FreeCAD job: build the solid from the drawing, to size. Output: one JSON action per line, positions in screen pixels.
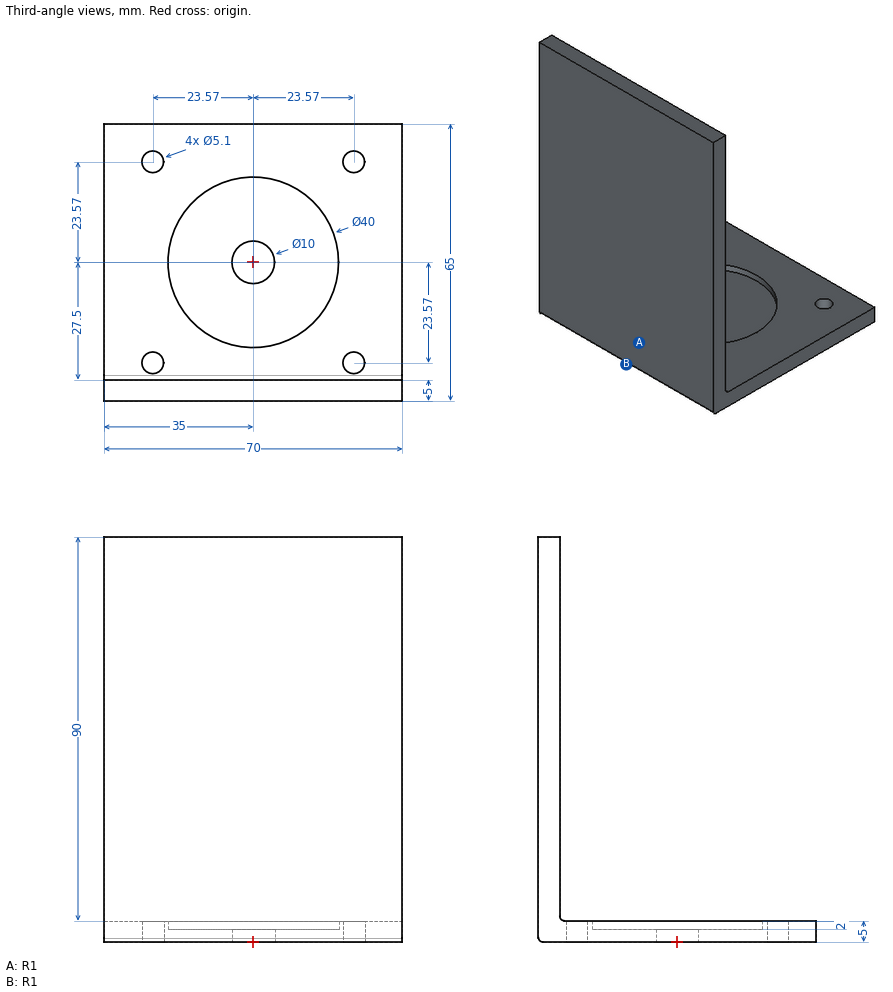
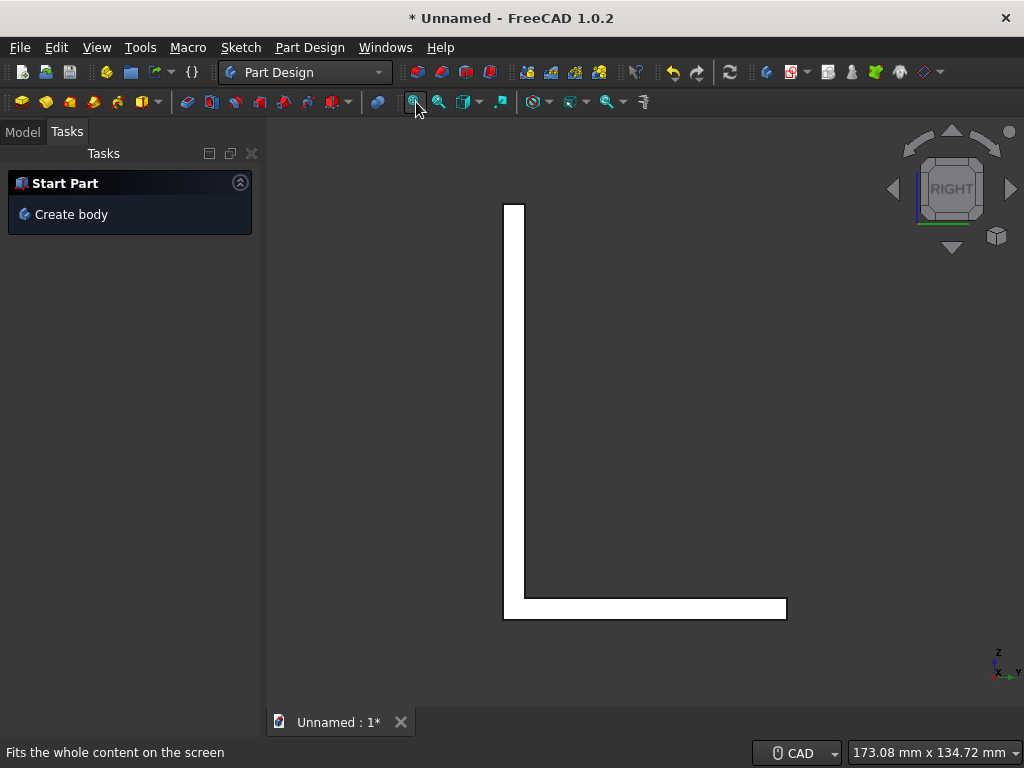
{"action": "key", "text": "5"}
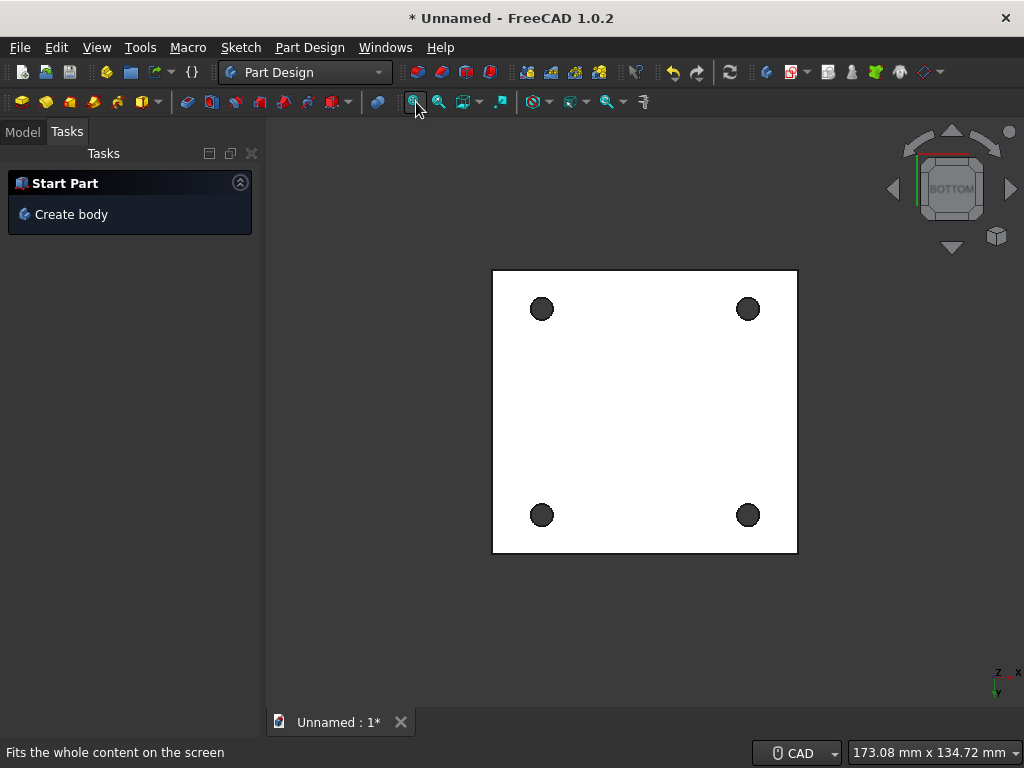
{"action": "key", "text": "4"}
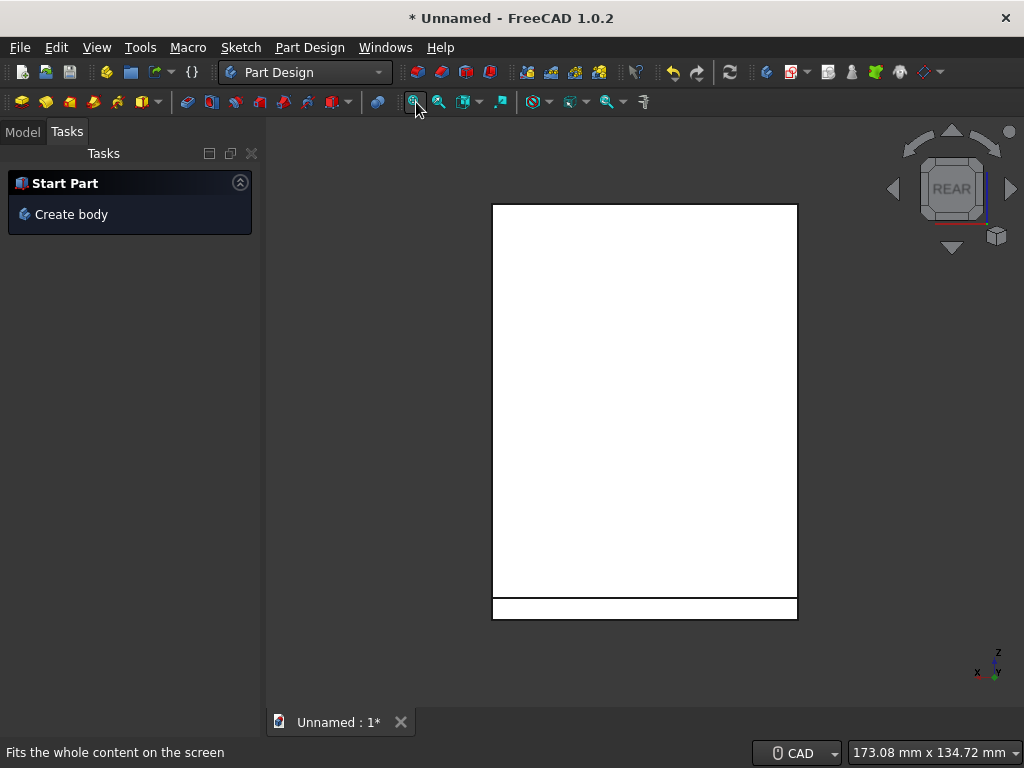
{"action": "key", "text": "6"}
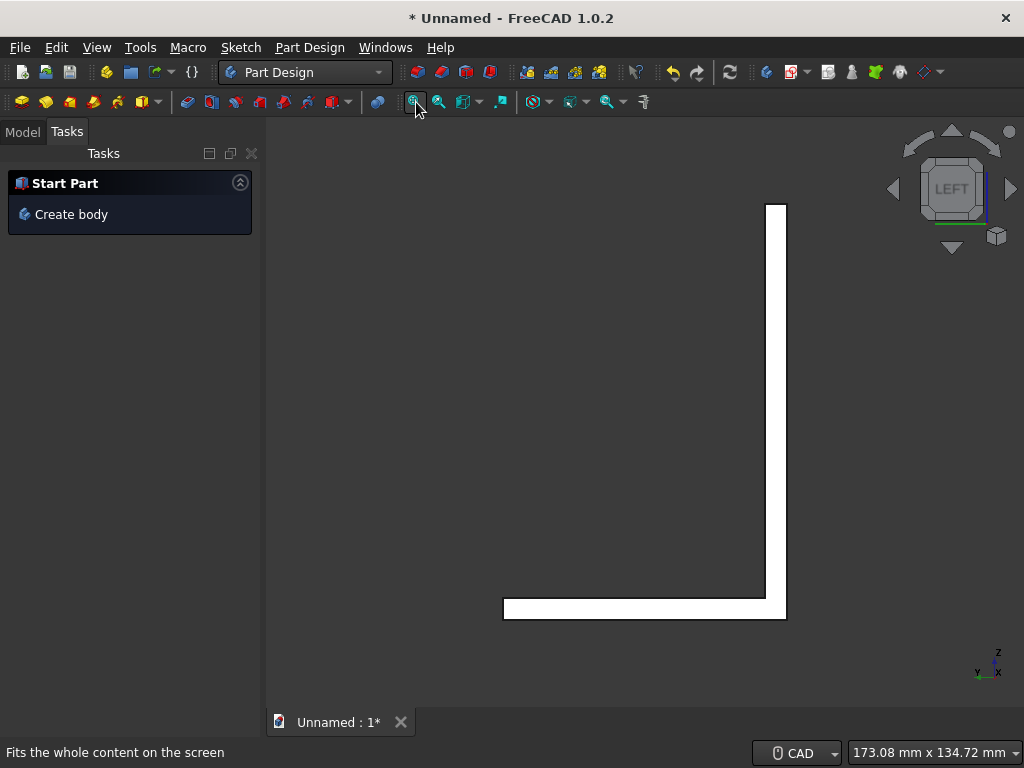
{"action": "key", "text": "v 3"}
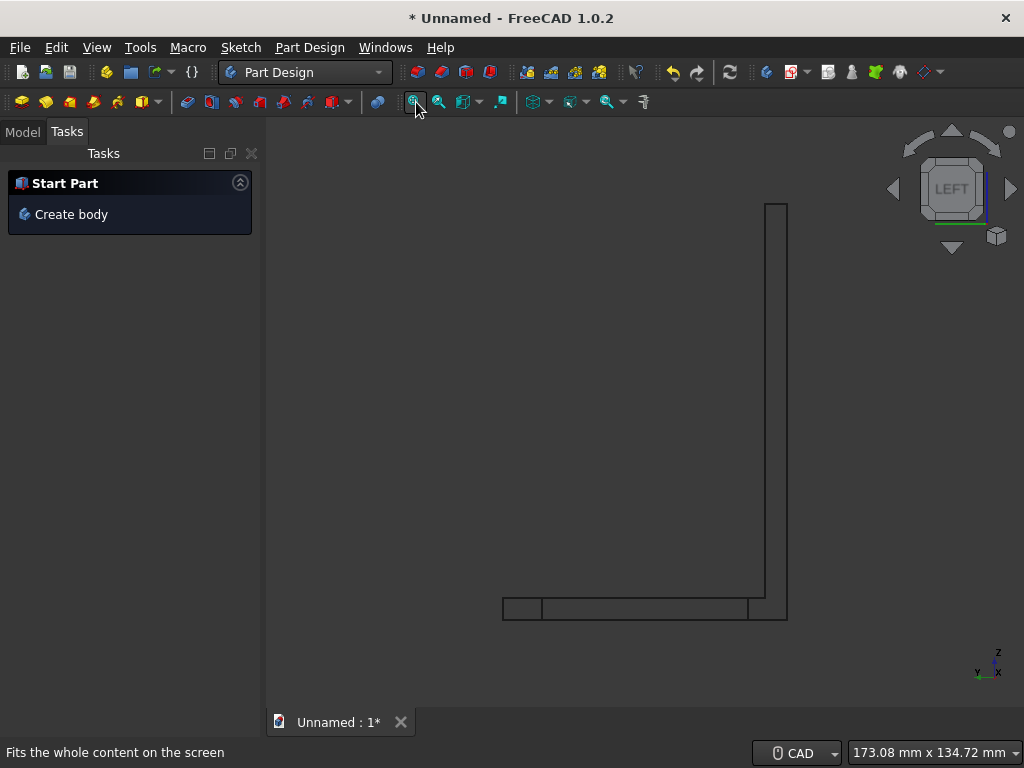
{"action": "key", "text": "0"}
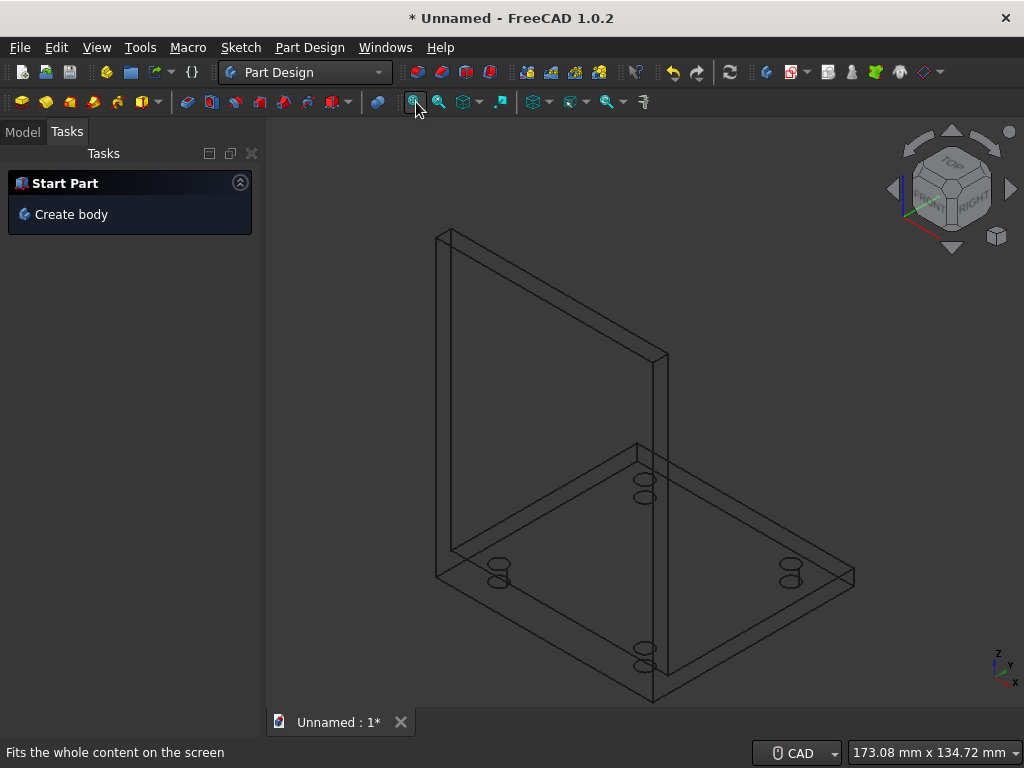
{"action": "left_click", "coordinate": [560, 612]}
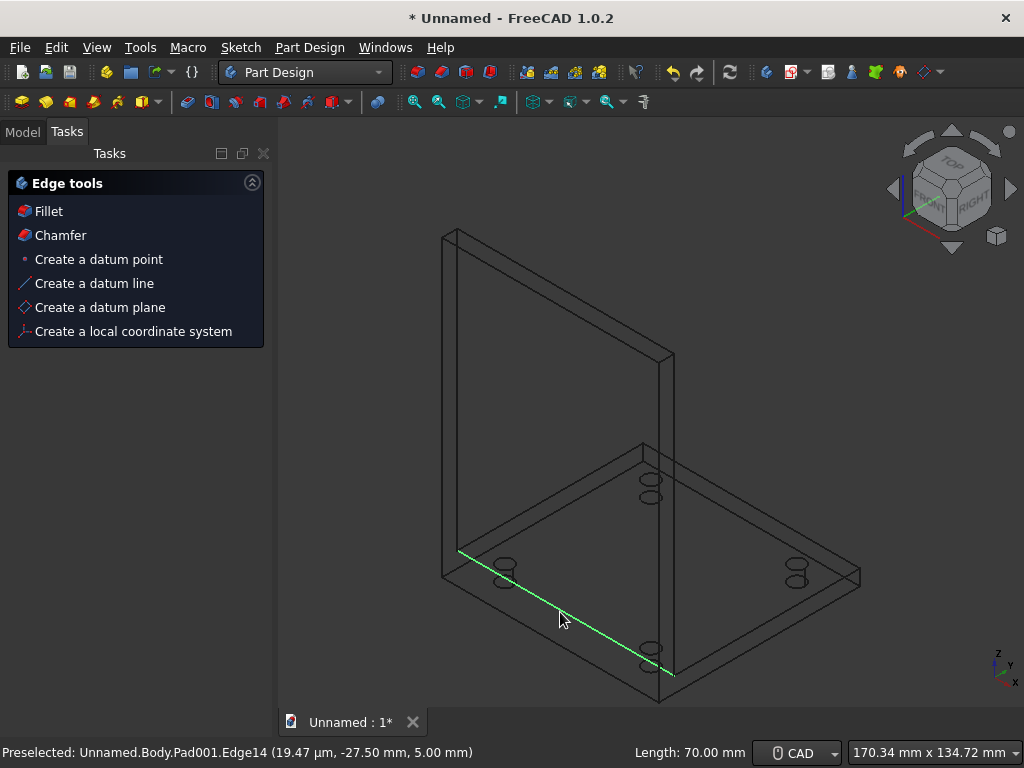
{"action": "key", "text": "v 1"}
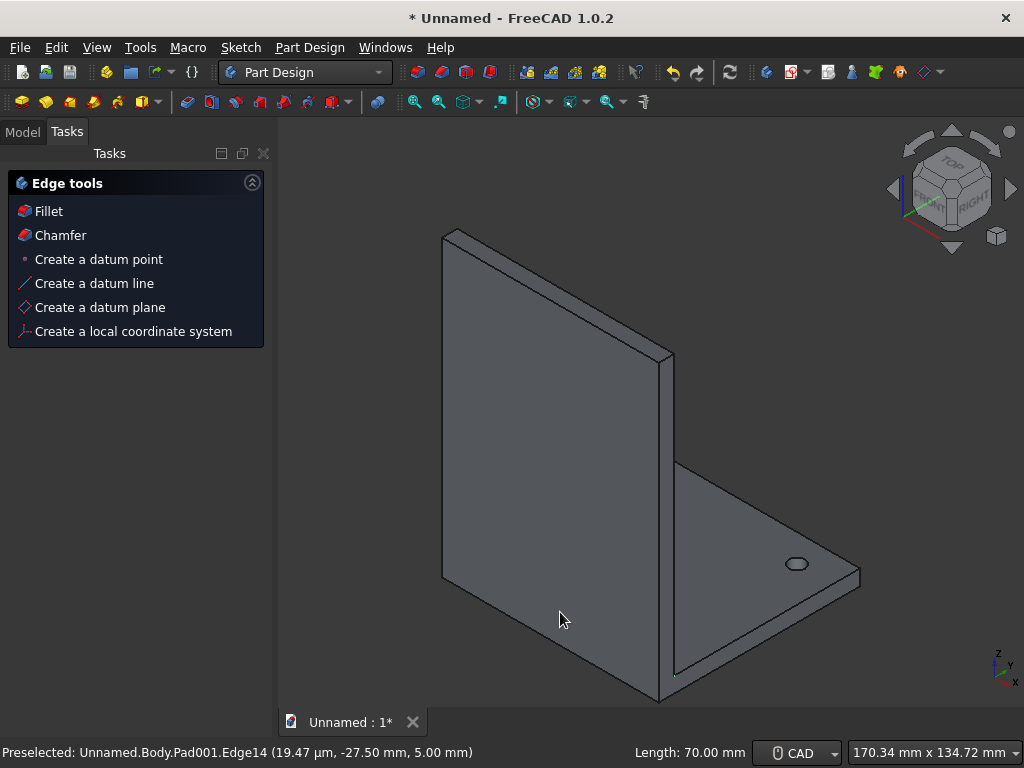
{"action": "left_click", "coordinate": [418, 72]}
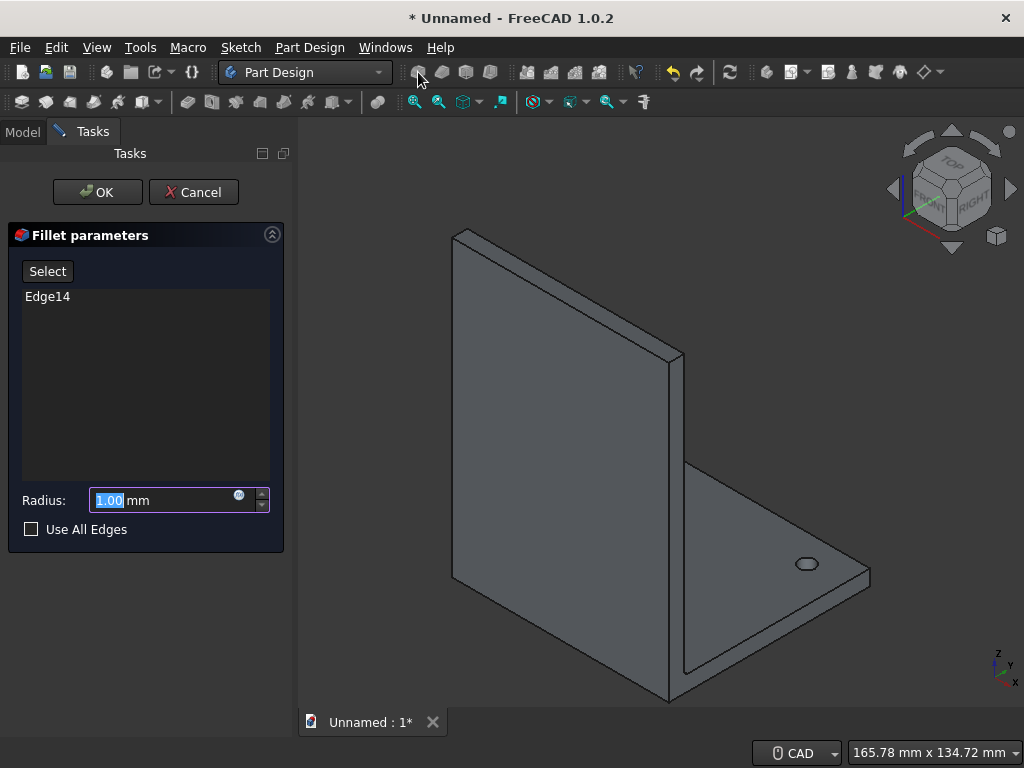
{"action": "type", "text": "1"}
{"action": "key", "text": "Tab"}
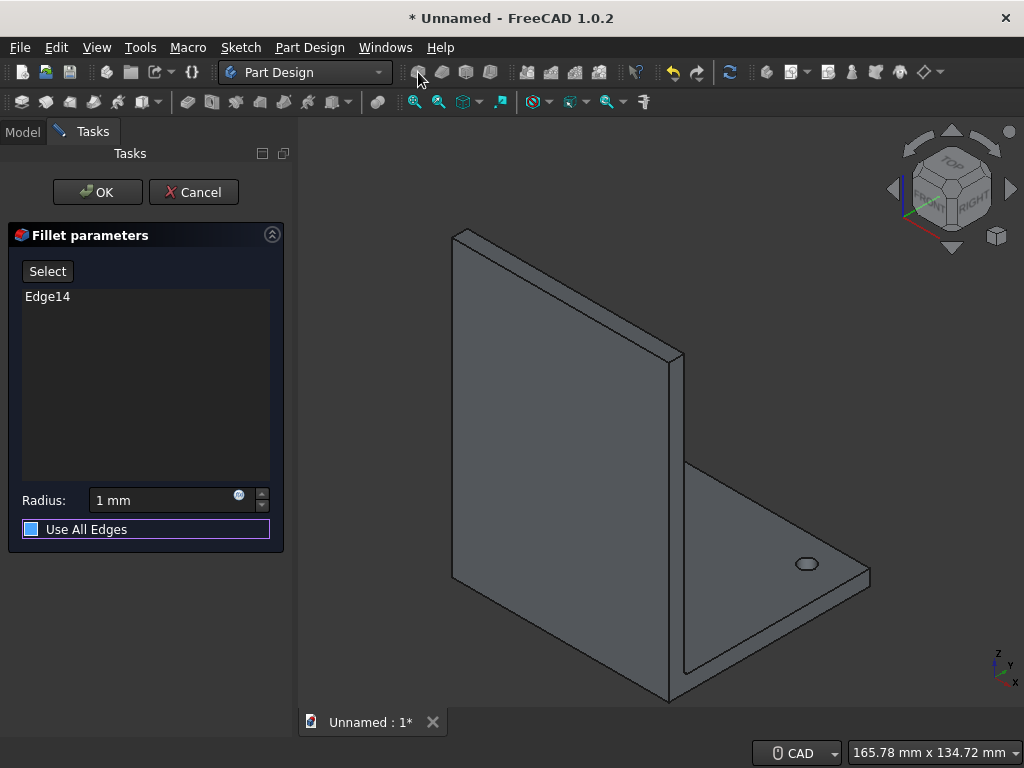
{"action": "left_click", "coordinate": [98, 192]}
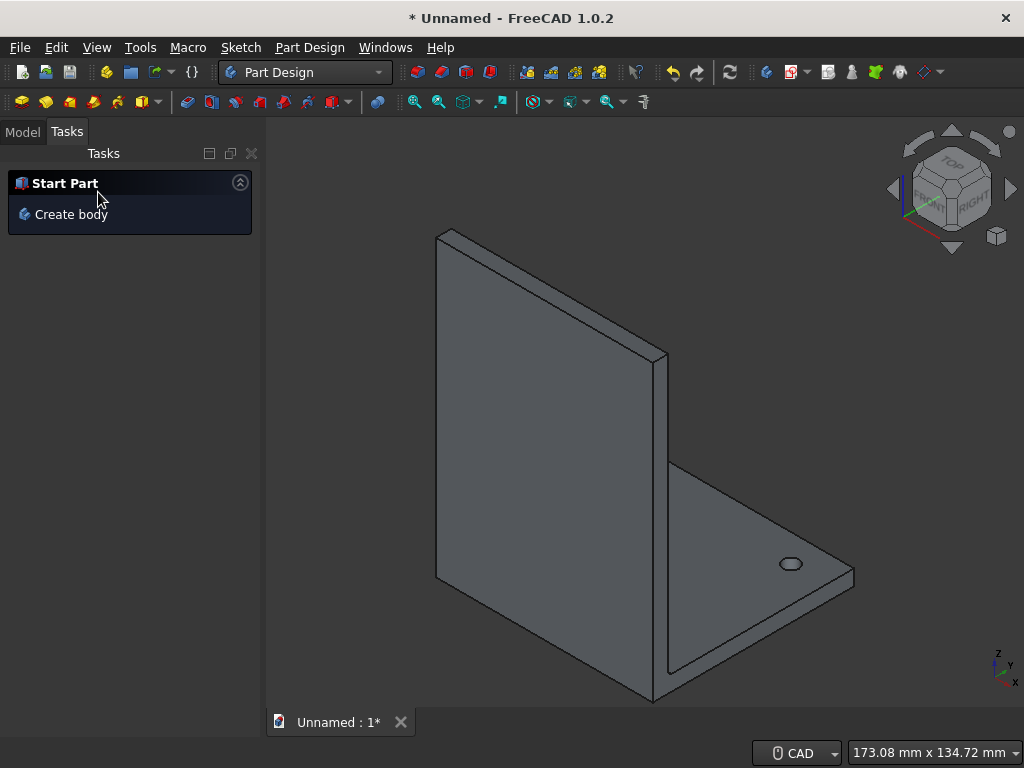
{"action": "key", "text": "2"}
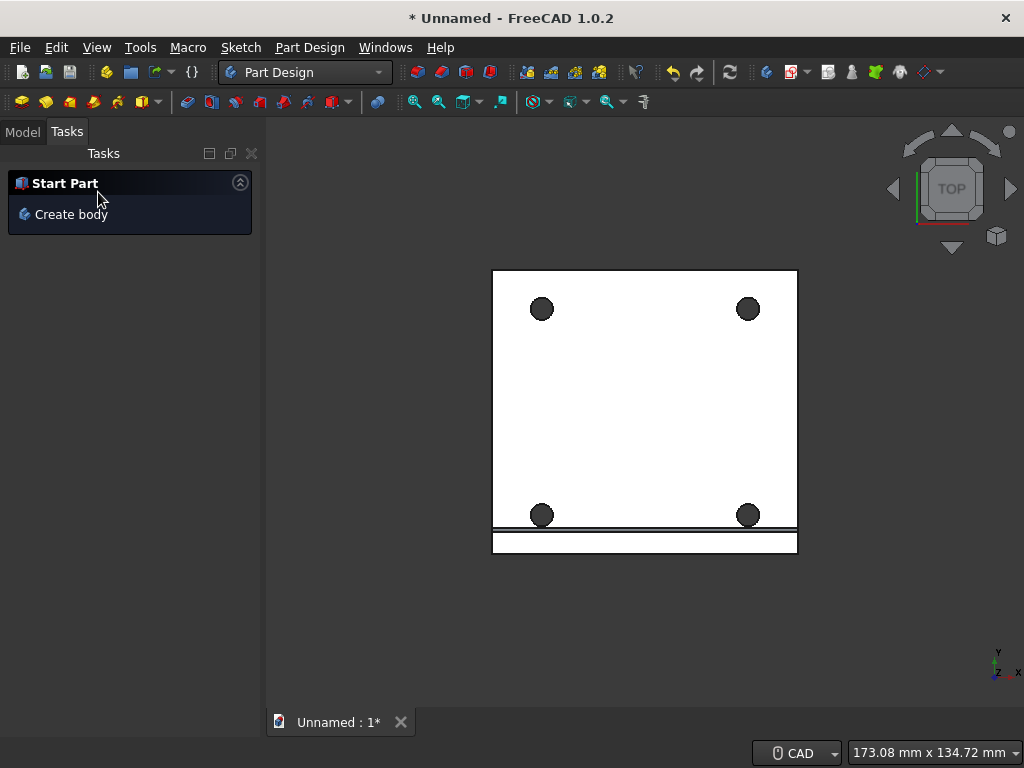
{"action": "key", "text": "0"}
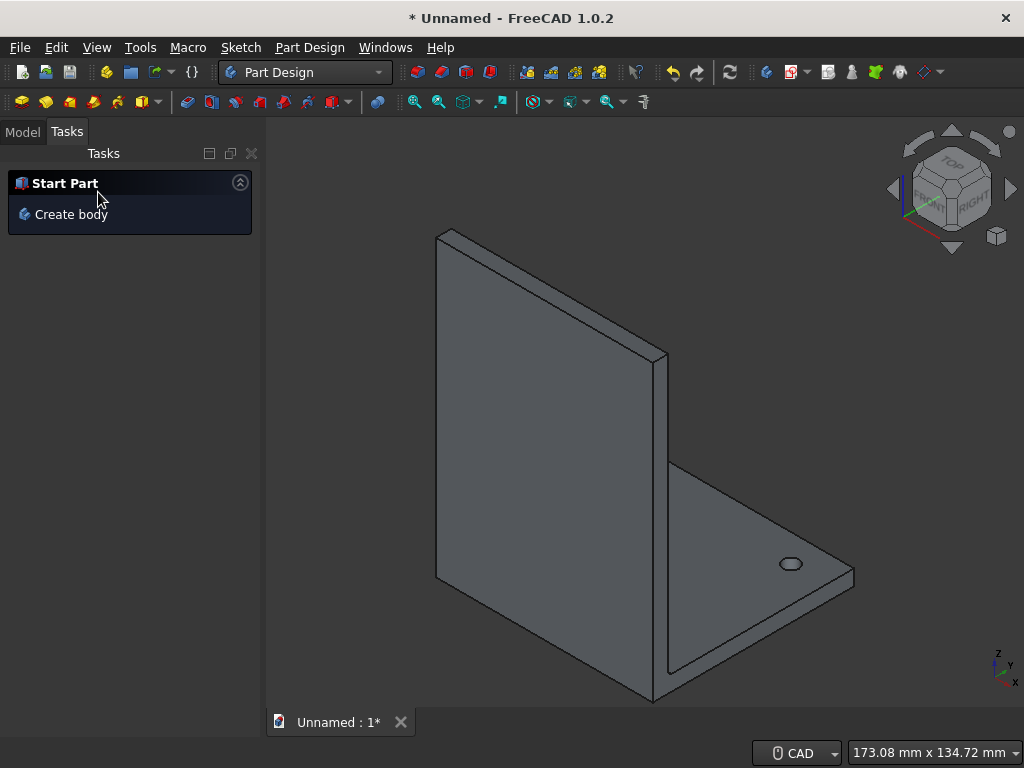
{"action": "key", "text": "1"}